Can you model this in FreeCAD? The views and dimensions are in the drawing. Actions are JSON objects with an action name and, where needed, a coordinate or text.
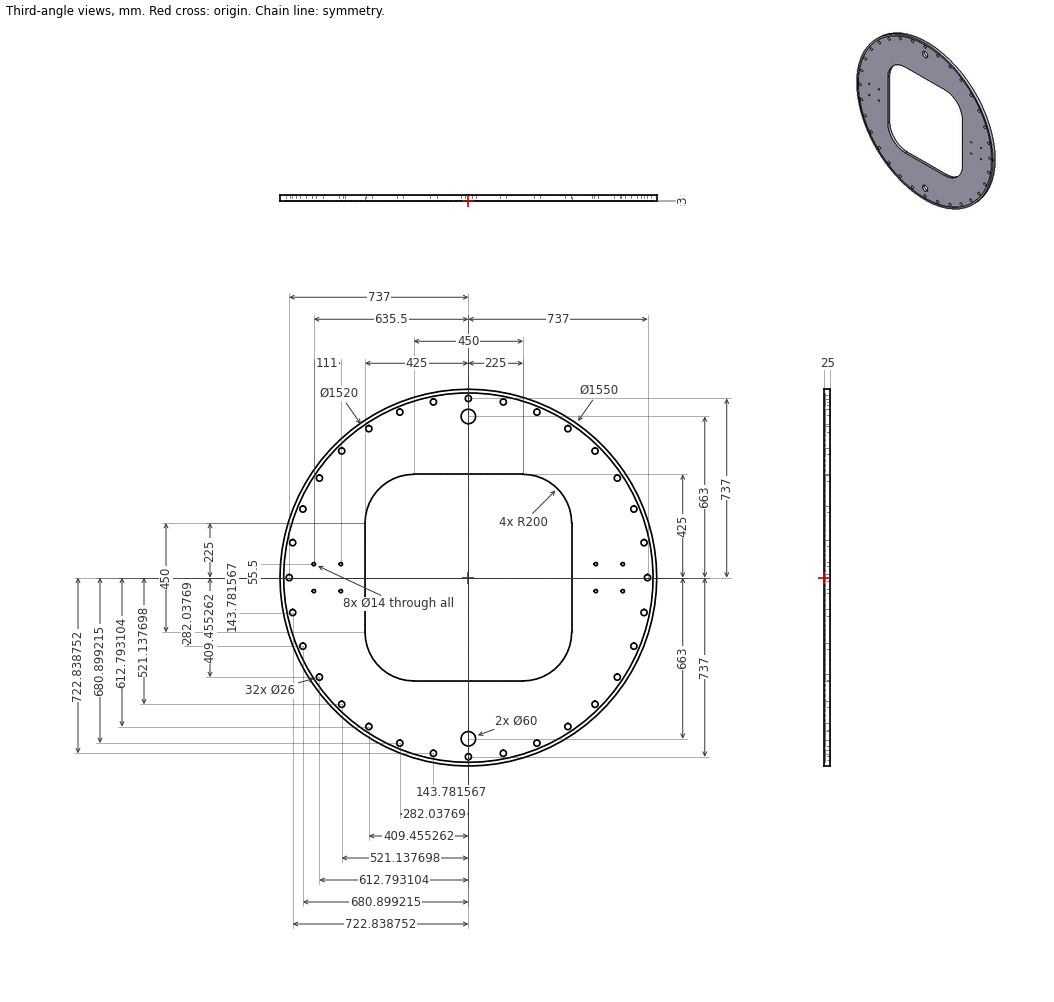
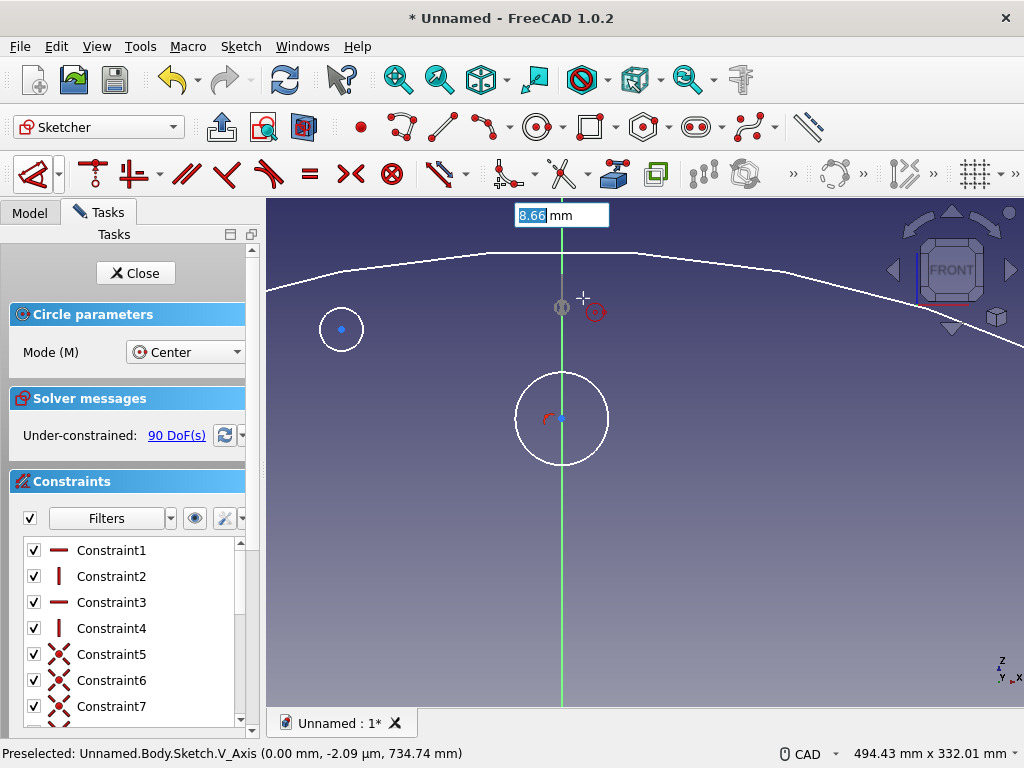
{"action": "left_click", "coordinate": [581, 297]}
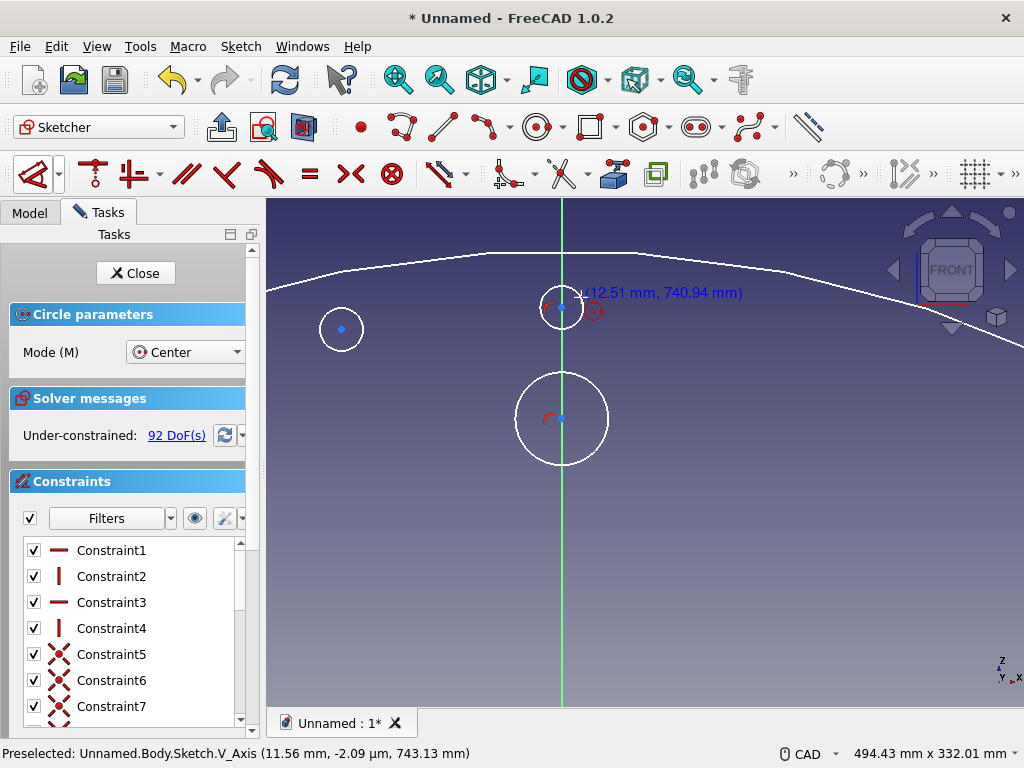
{"action": "scroll", "coordinate": [579, 299], "scroll_direction": "down", "scroll_amount": 10}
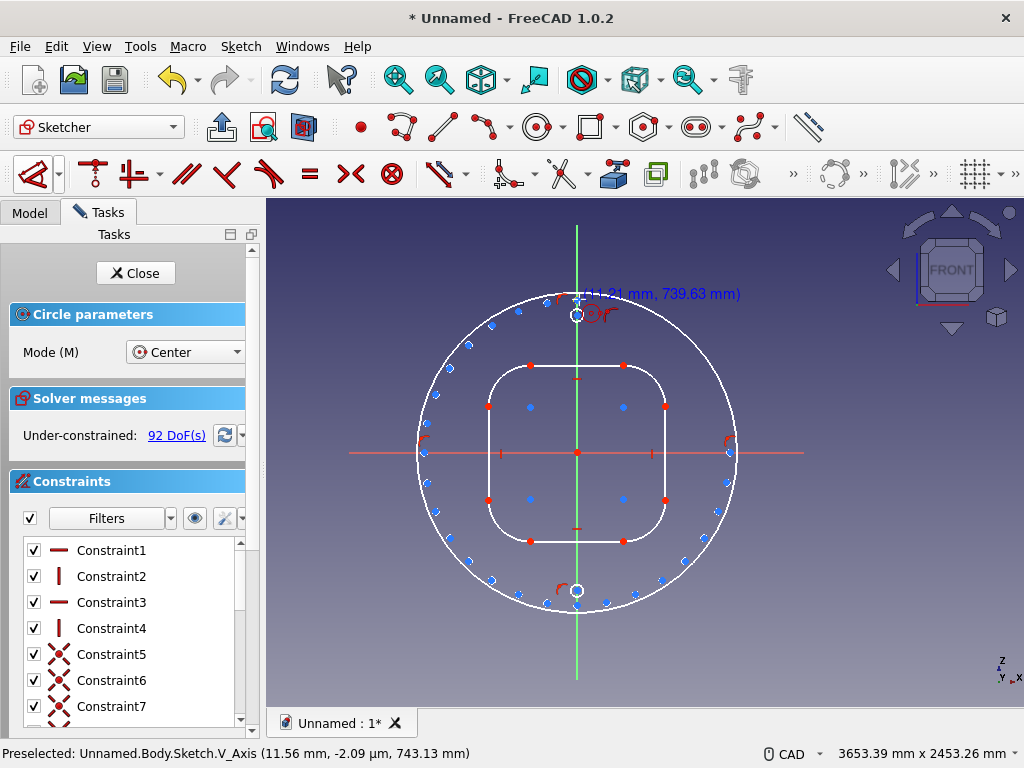
{"action": "scroll", "coordinate": [607, 303], "scroll_direction": "up", "scroll_amount": 4}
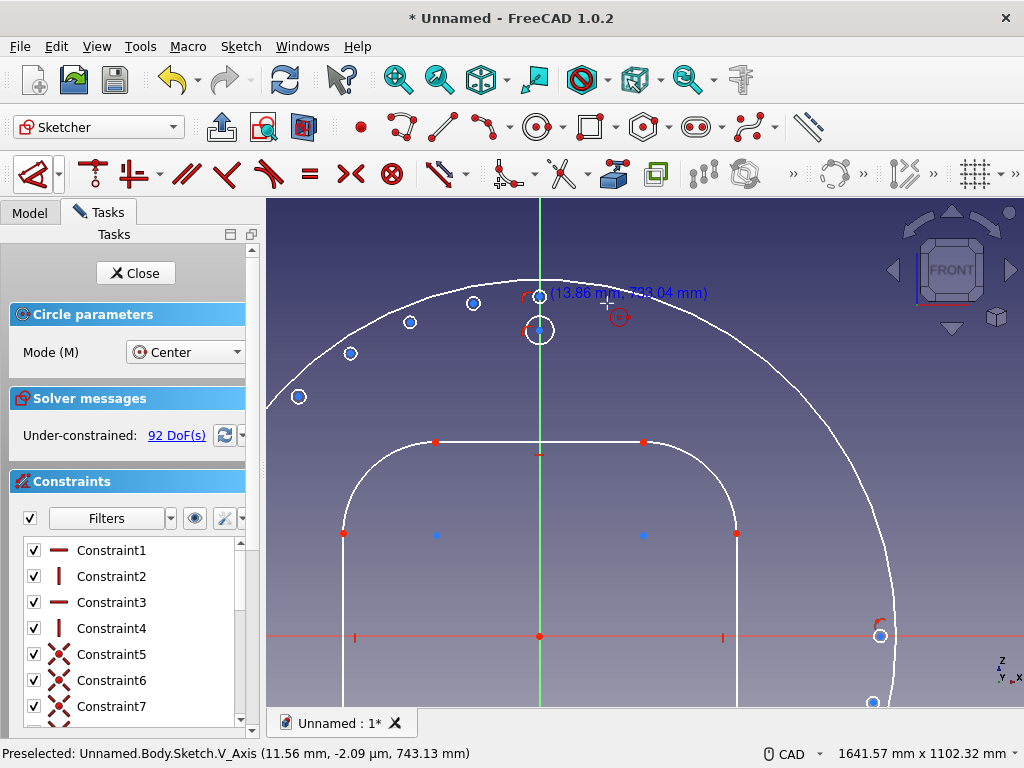
{"action": "left_click", "coordinate": [606, 302]}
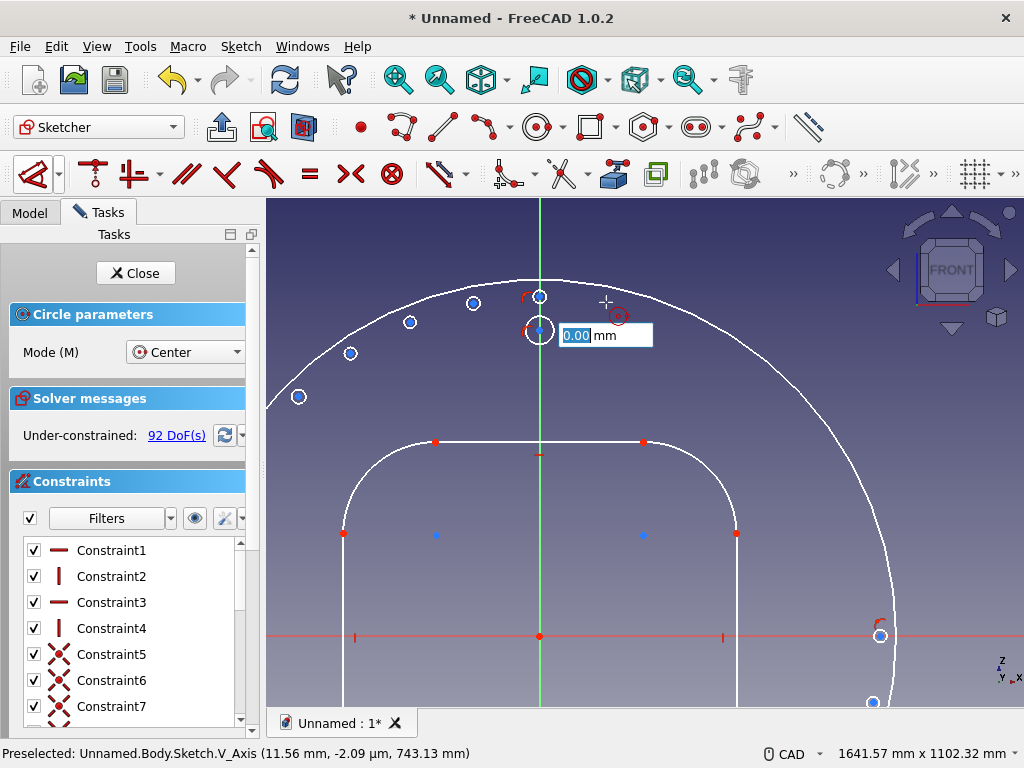
{"action": "scroll", "coordinate": [602, 298], "scroll_direction": "up", "scroll_amount": 5}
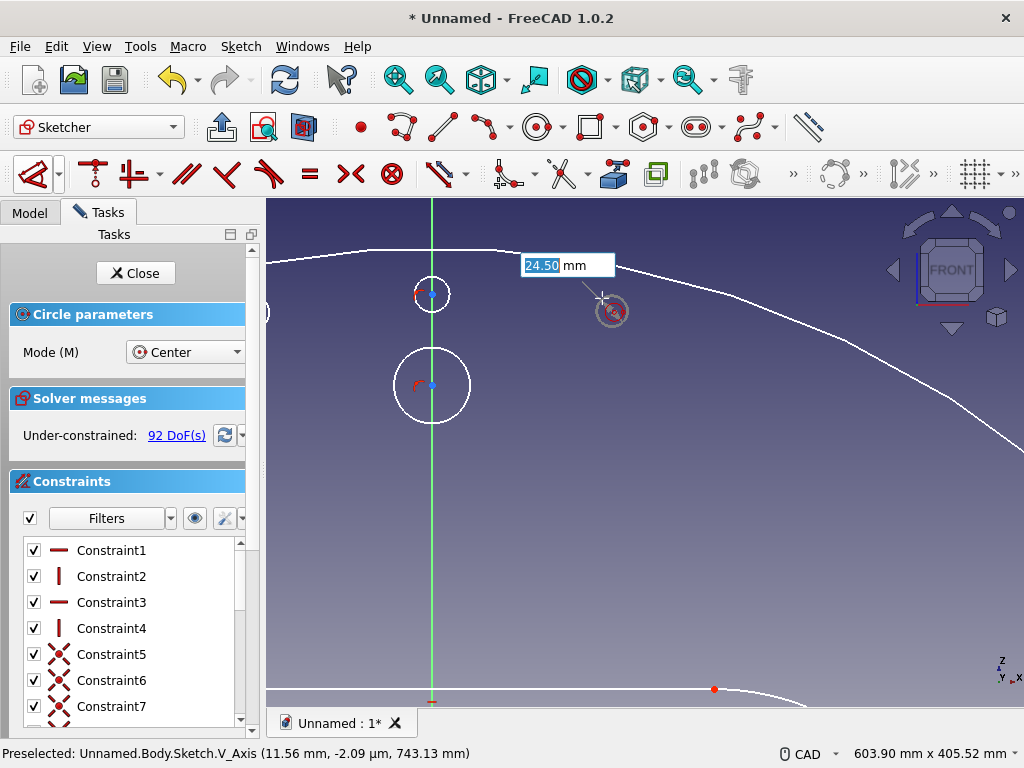
{"action": "left_click", "coordinate": [601, 298]}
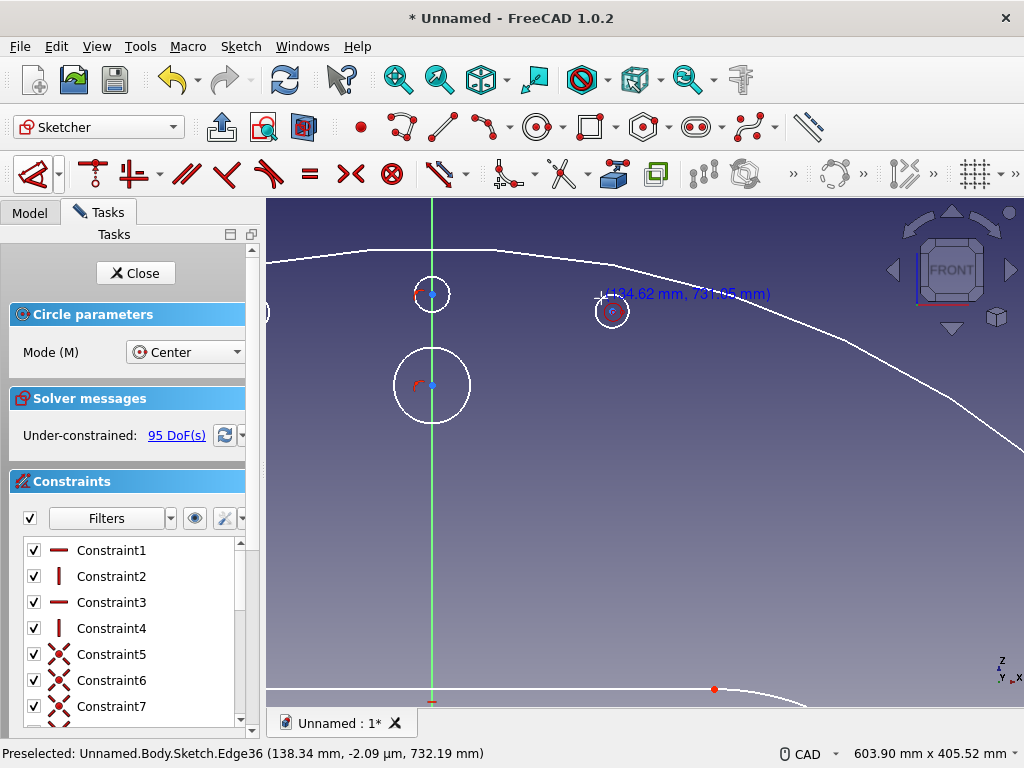
{"action": "scroll", "coordinate": [786, 362], "scroll_direction": "up", "scroll_amount": 2}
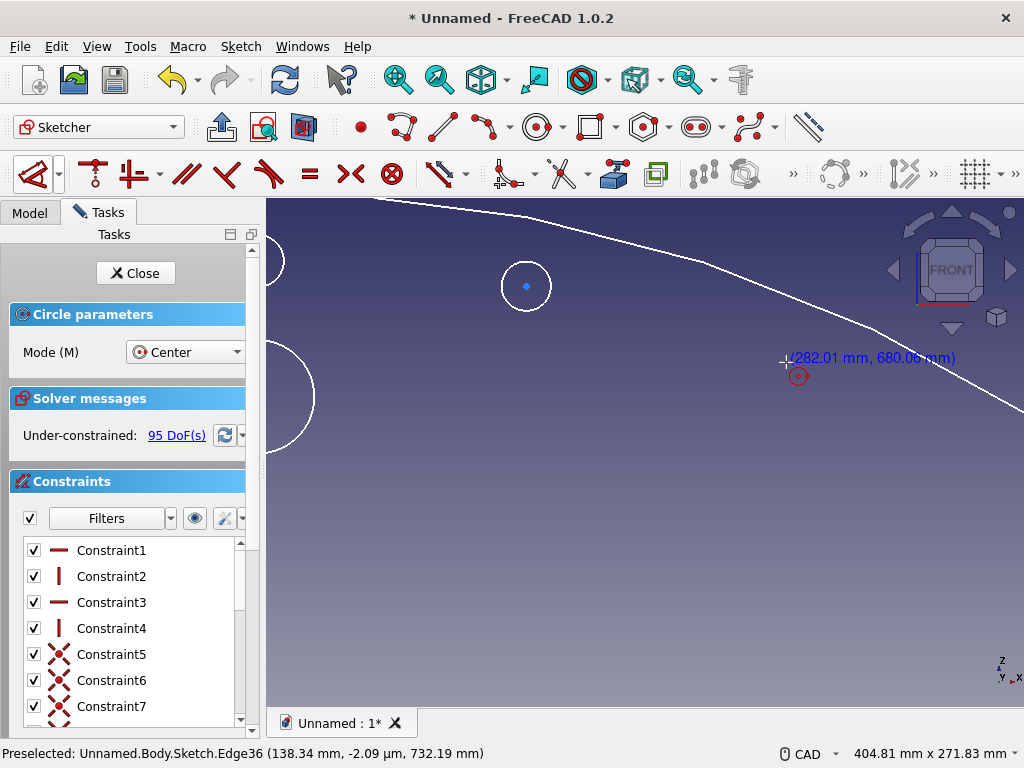
{"action": "scroll", "coordinate": [616, 305], "scroll_direction": "down", "scroll_amount": 11}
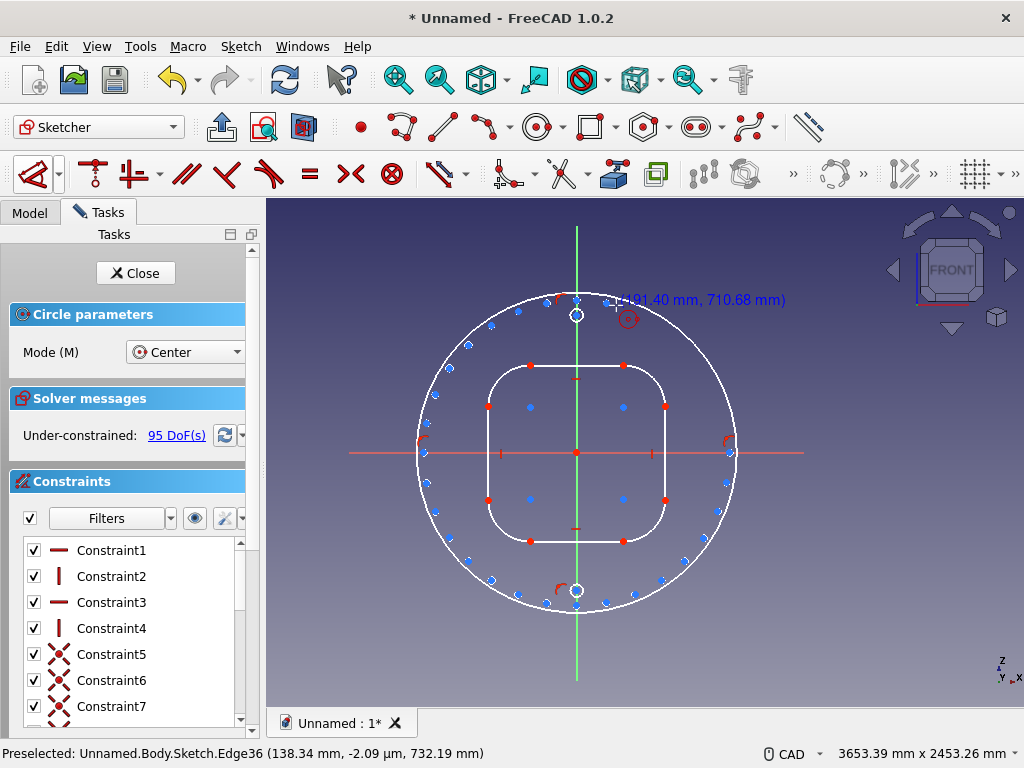
{"action": "scroll", "coordinate": [635, 311], "scroll_direction": "up", "scroll_amount": 4}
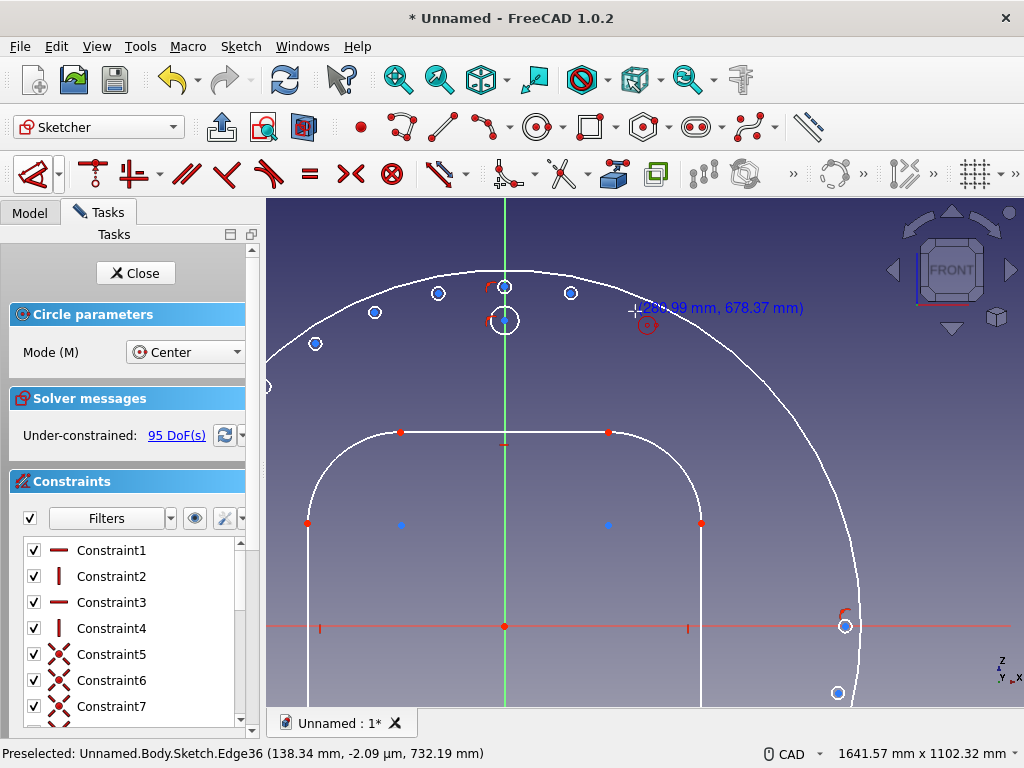
{"action": "left_click", "coordinate": [635, 312]}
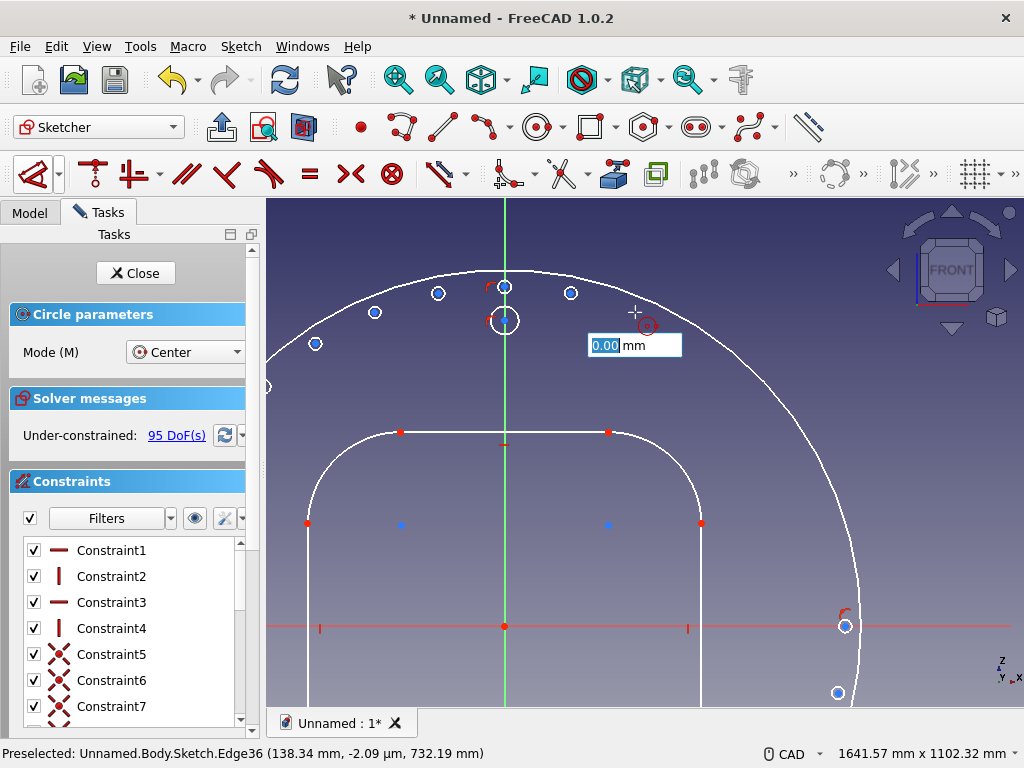
{"action": "scroll", "coordinate": [631, 308], "scroll_direction": "up", "scroll_amount": 5}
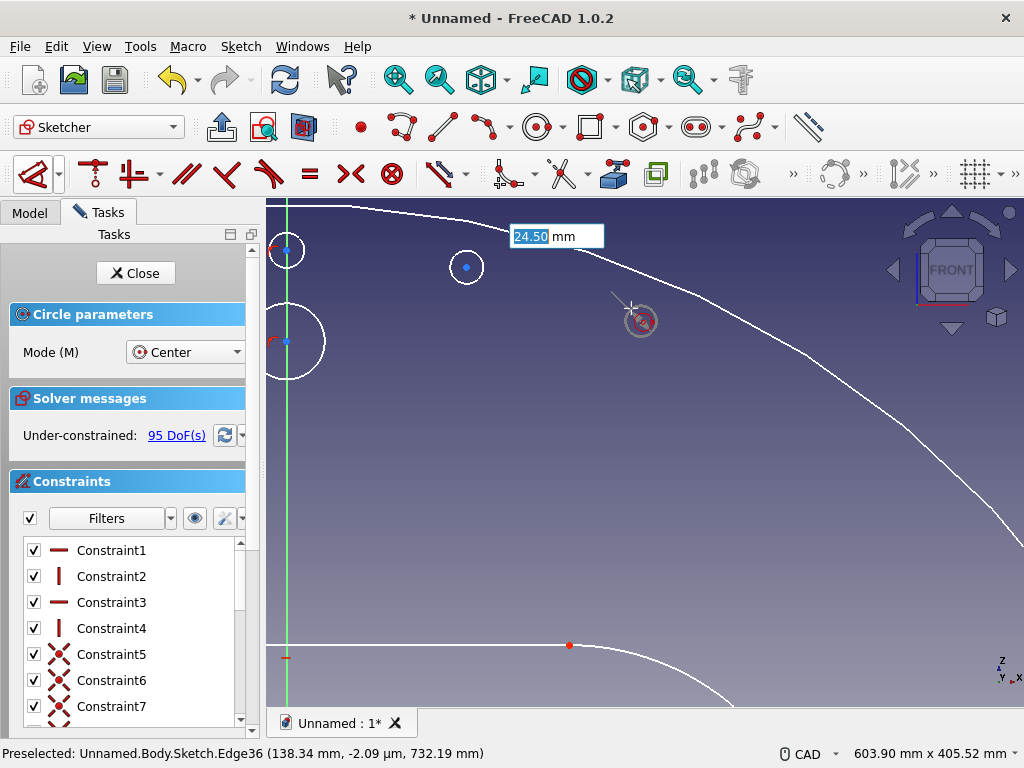
{"action": "left_click", "coordinate": [629, 306]}